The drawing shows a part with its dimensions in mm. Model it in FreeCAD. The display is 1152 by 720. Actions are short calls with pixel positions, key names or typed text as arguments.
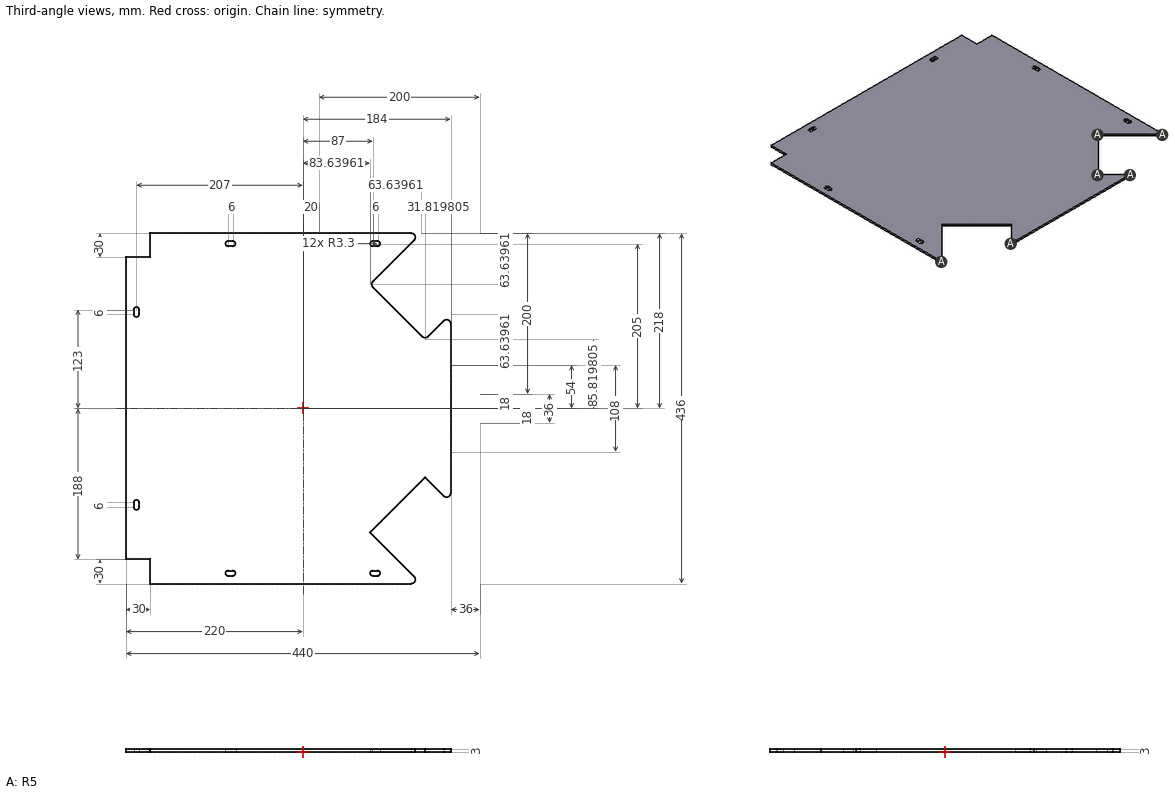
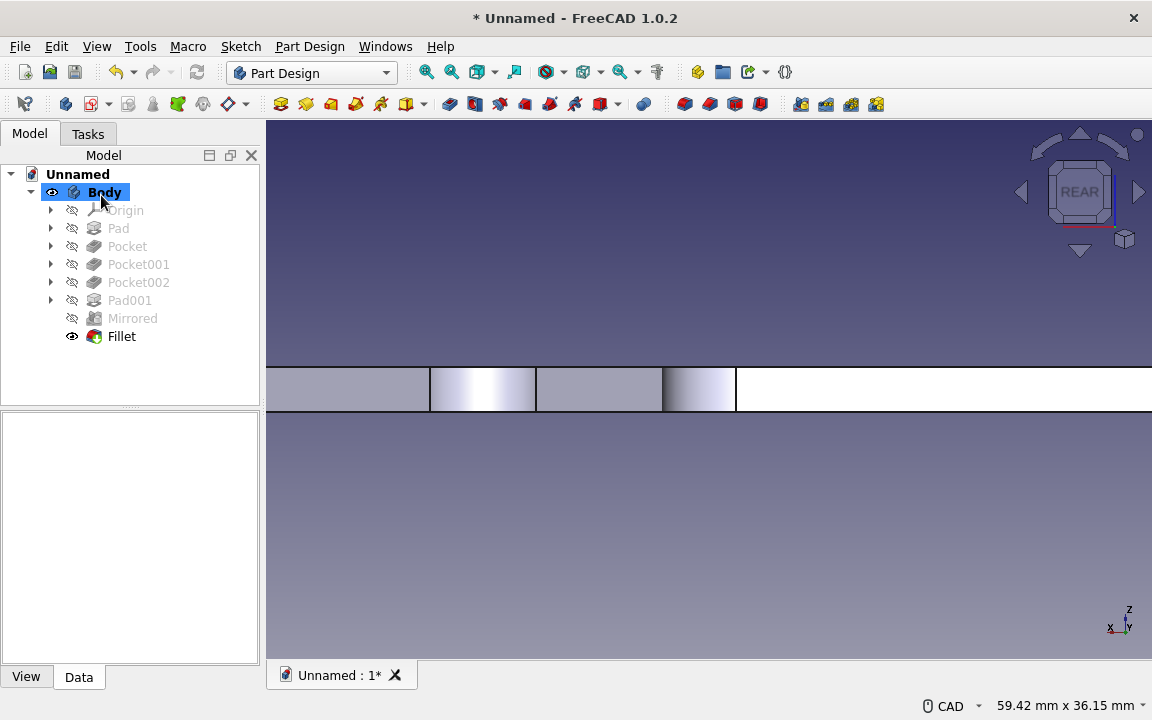
click(427, 72)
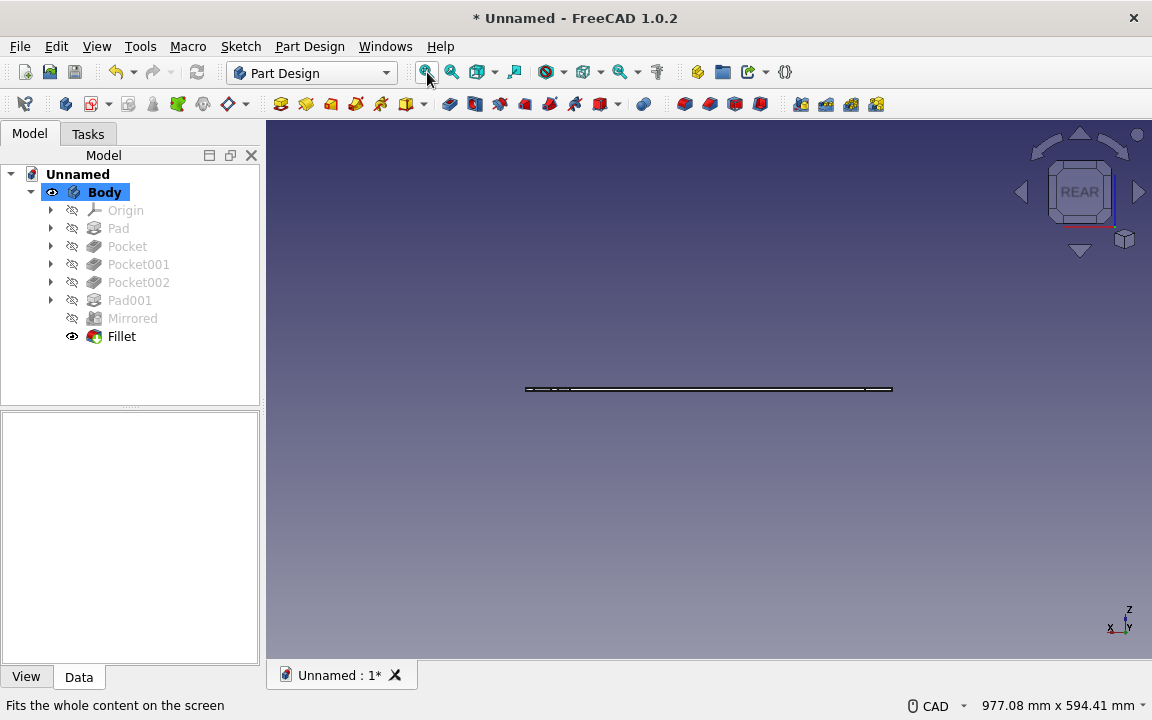
key(5)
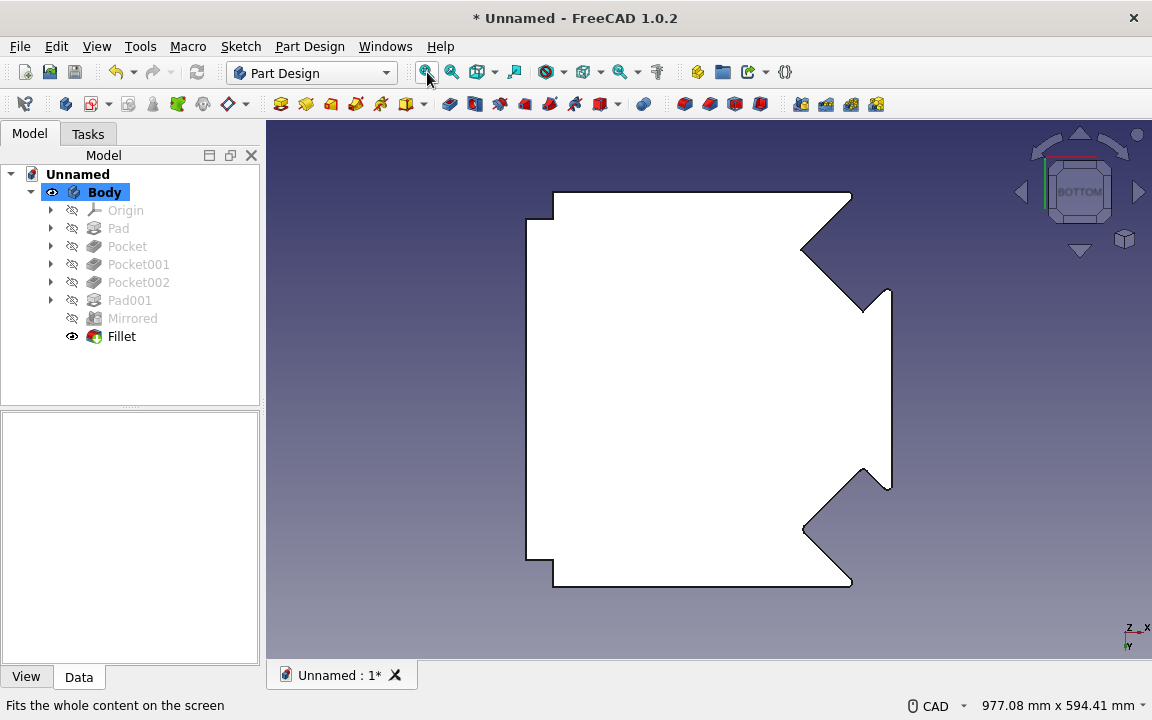
click(709, 388)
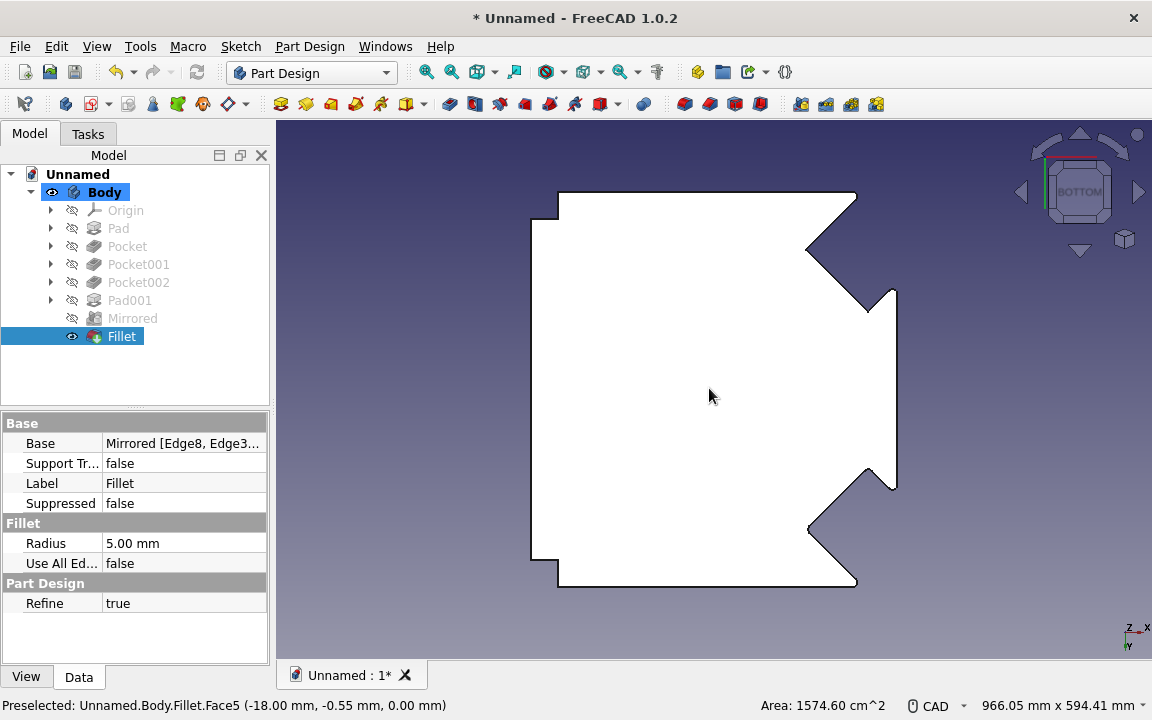
click(90, 104)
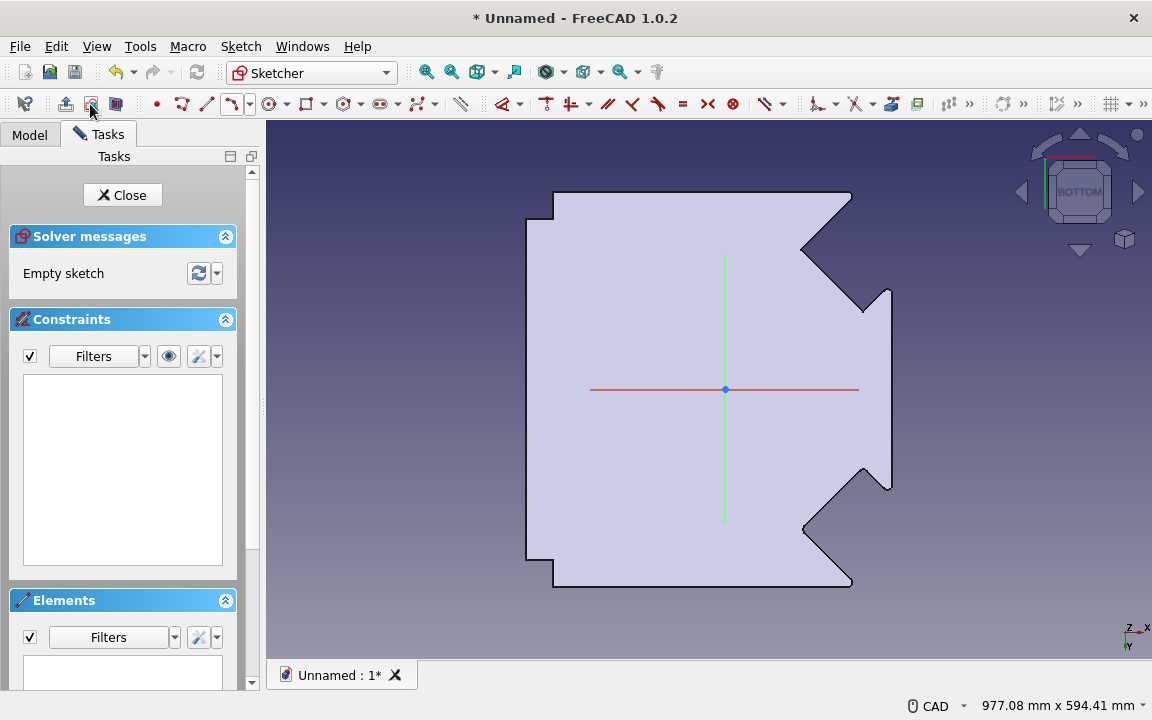
key(g)
key(s)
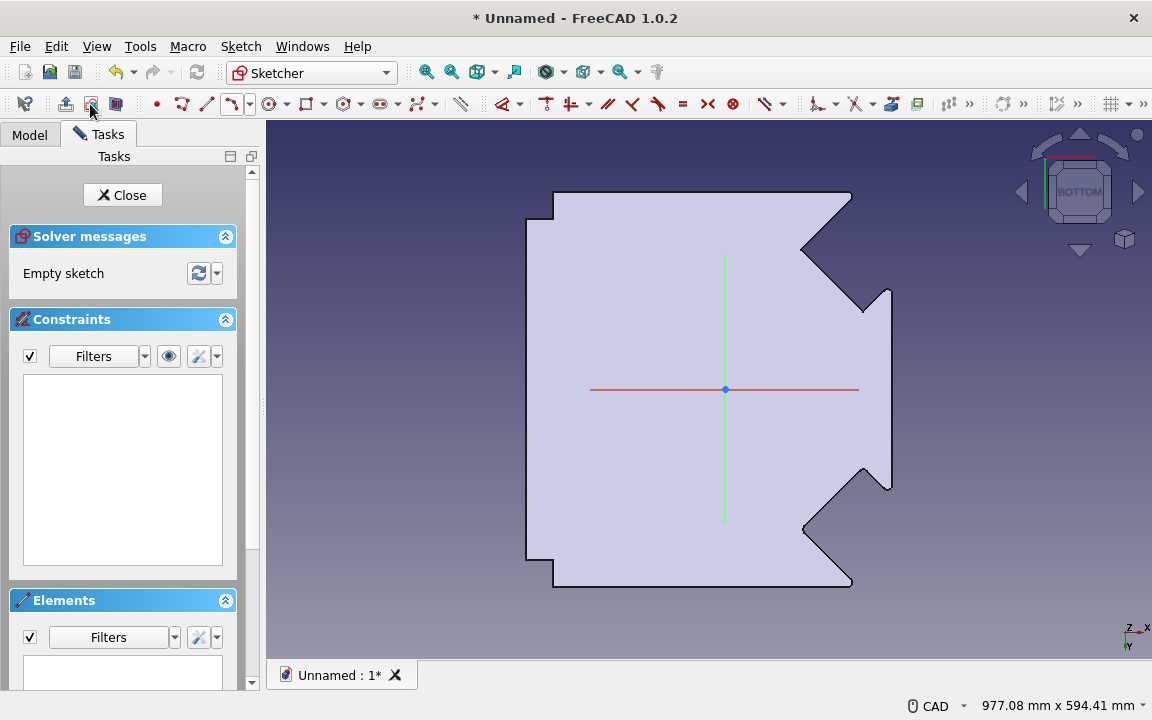
scroll(804, 575, up, 11)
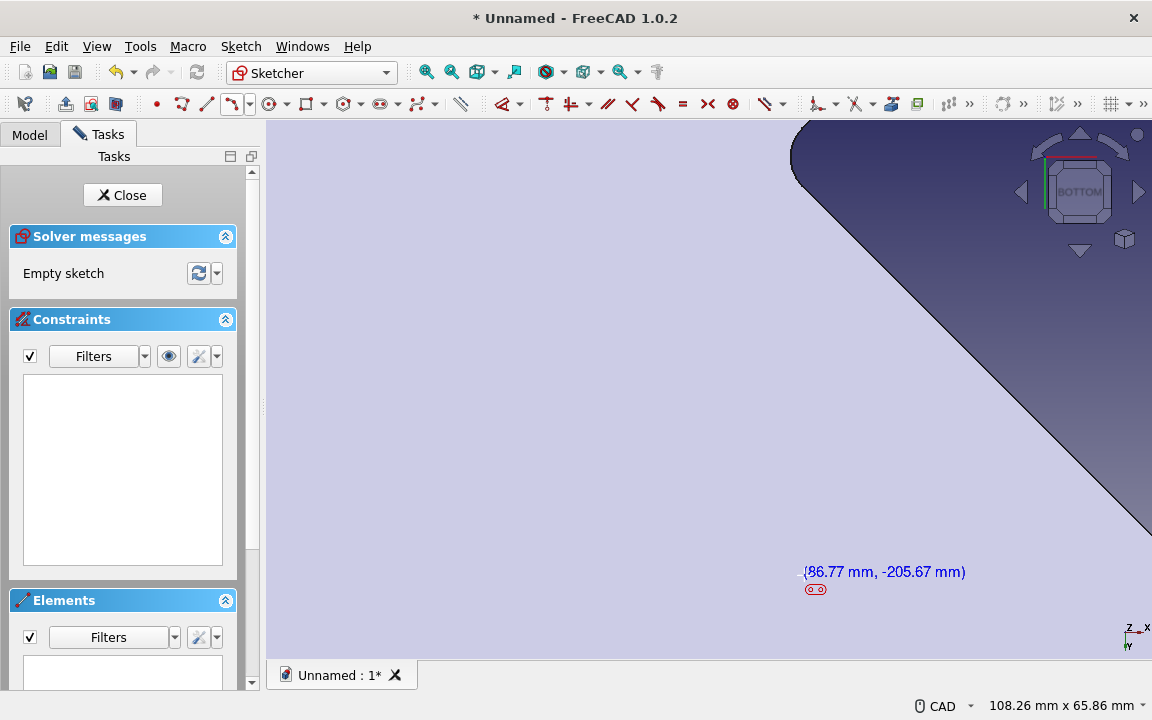
scroll(742, 539, down, 12)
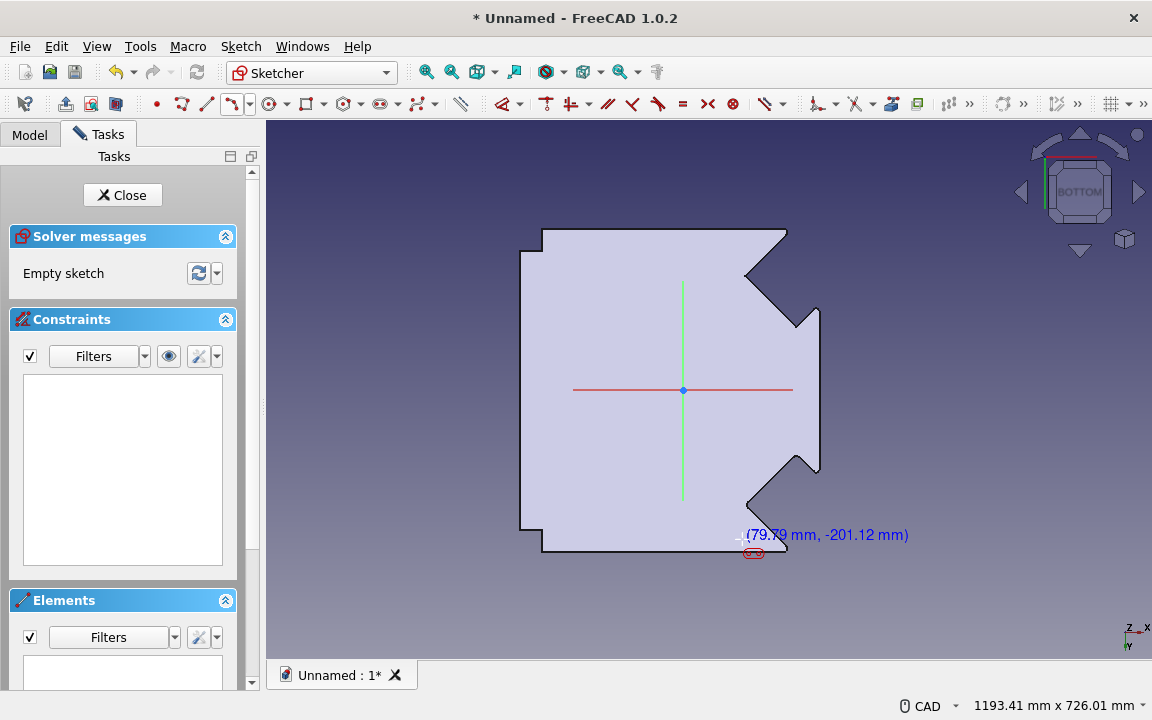
click(748, 543)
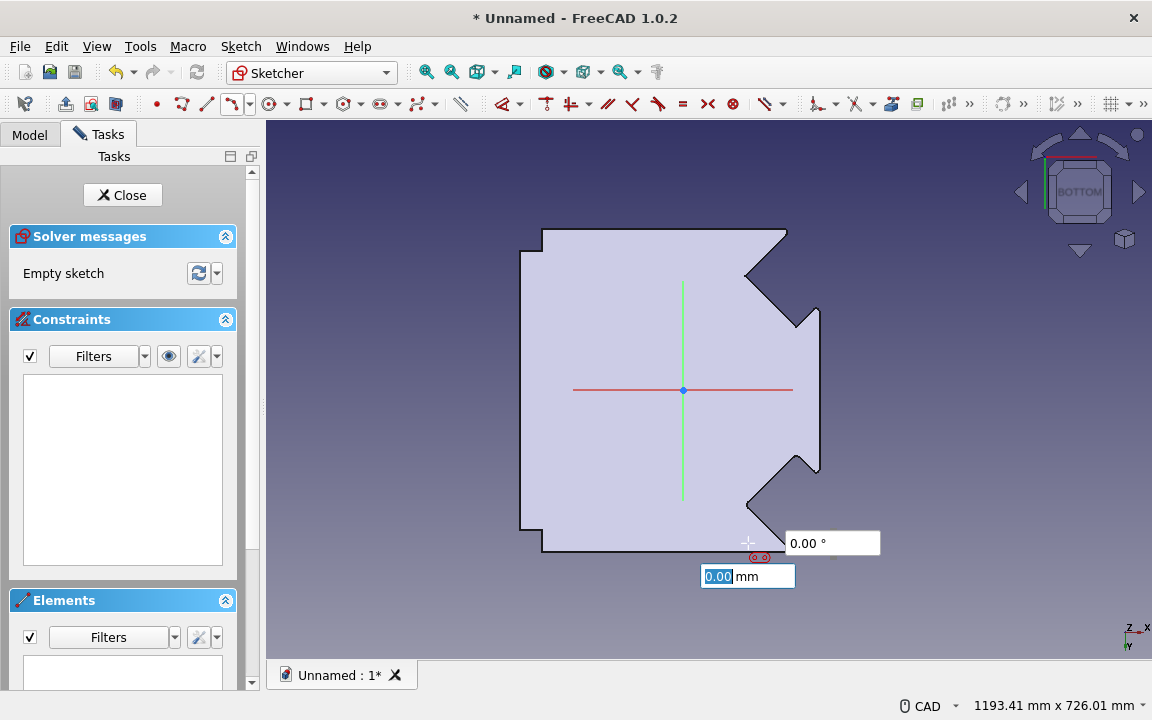
scroll(752, 543, up, 7)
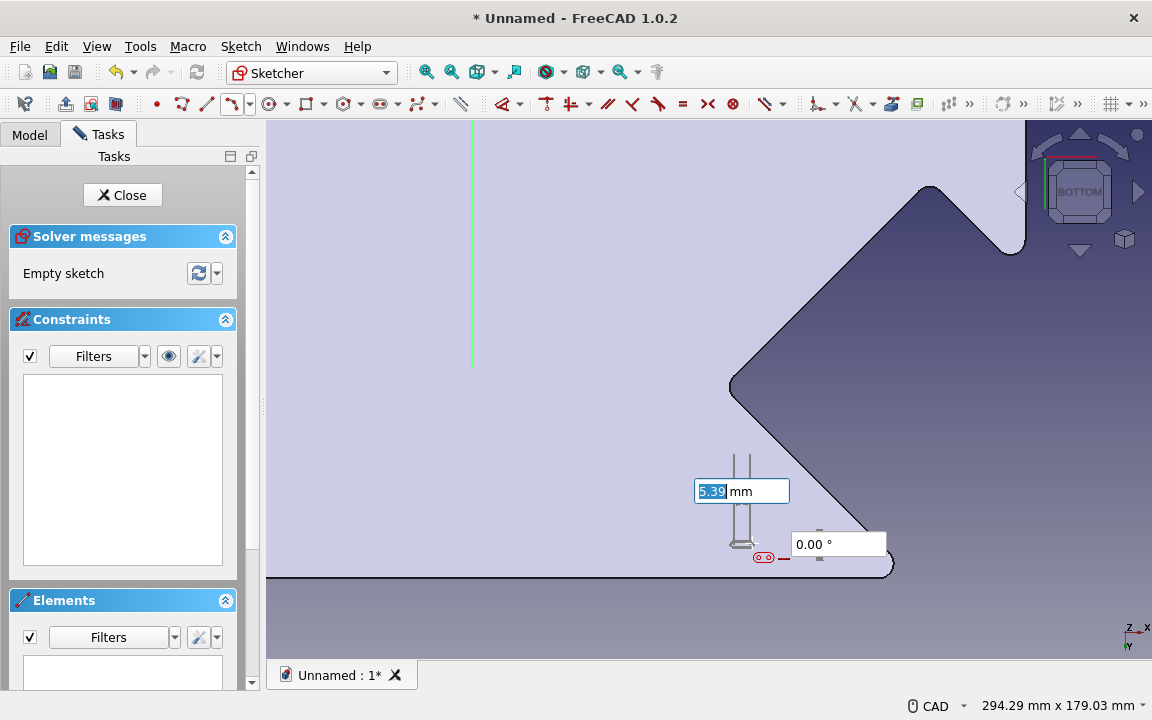
click(752, 541)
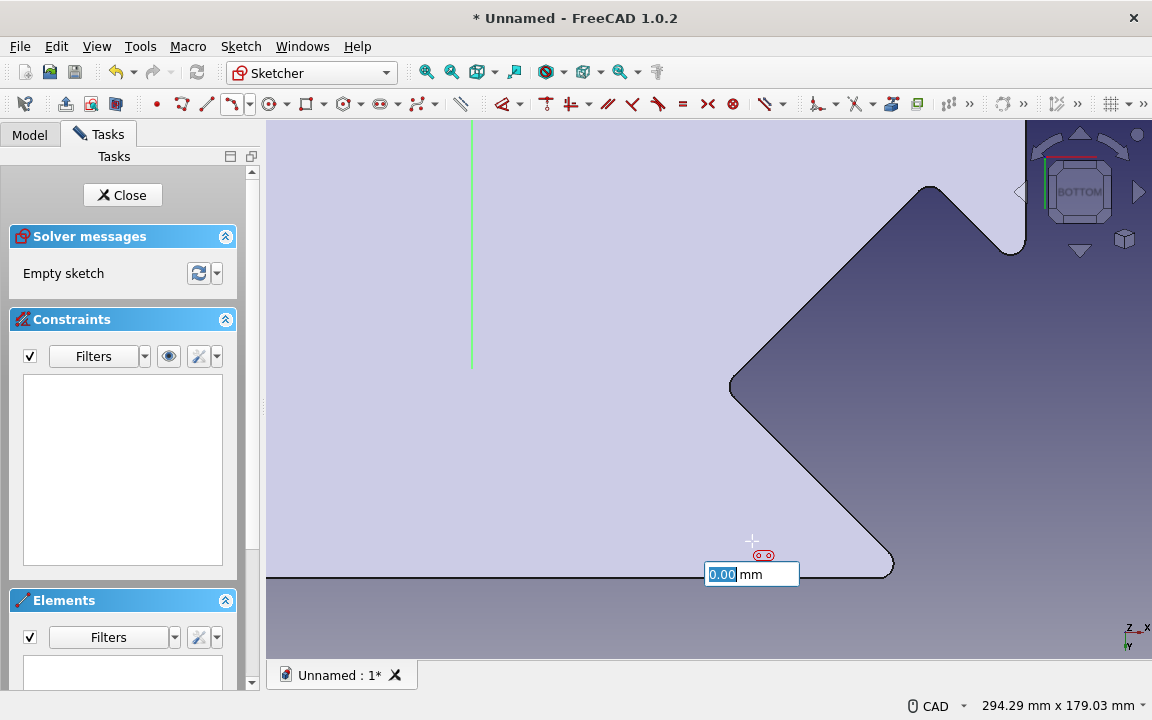
scroll(743, 549, up, 3)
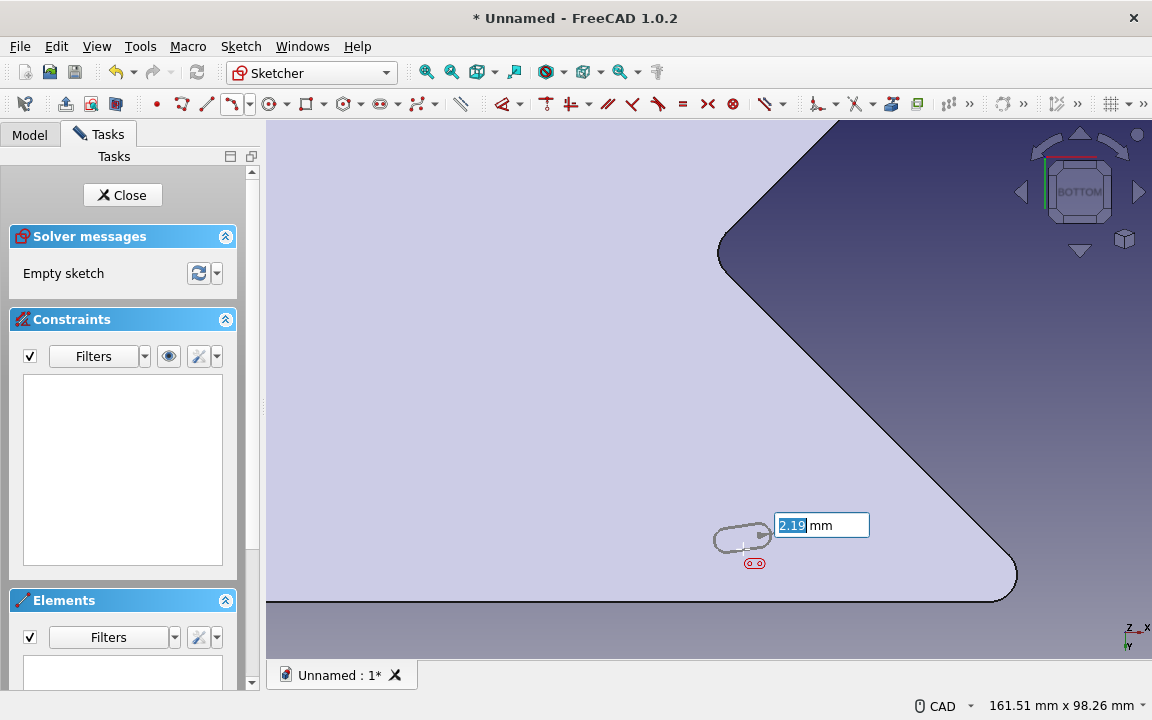
click(742, 549)